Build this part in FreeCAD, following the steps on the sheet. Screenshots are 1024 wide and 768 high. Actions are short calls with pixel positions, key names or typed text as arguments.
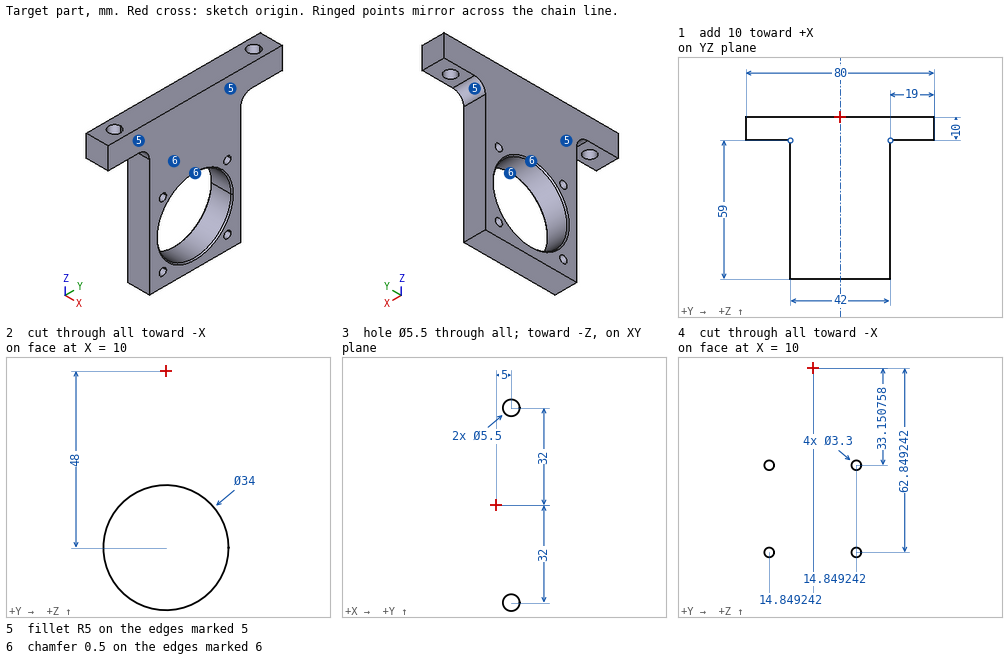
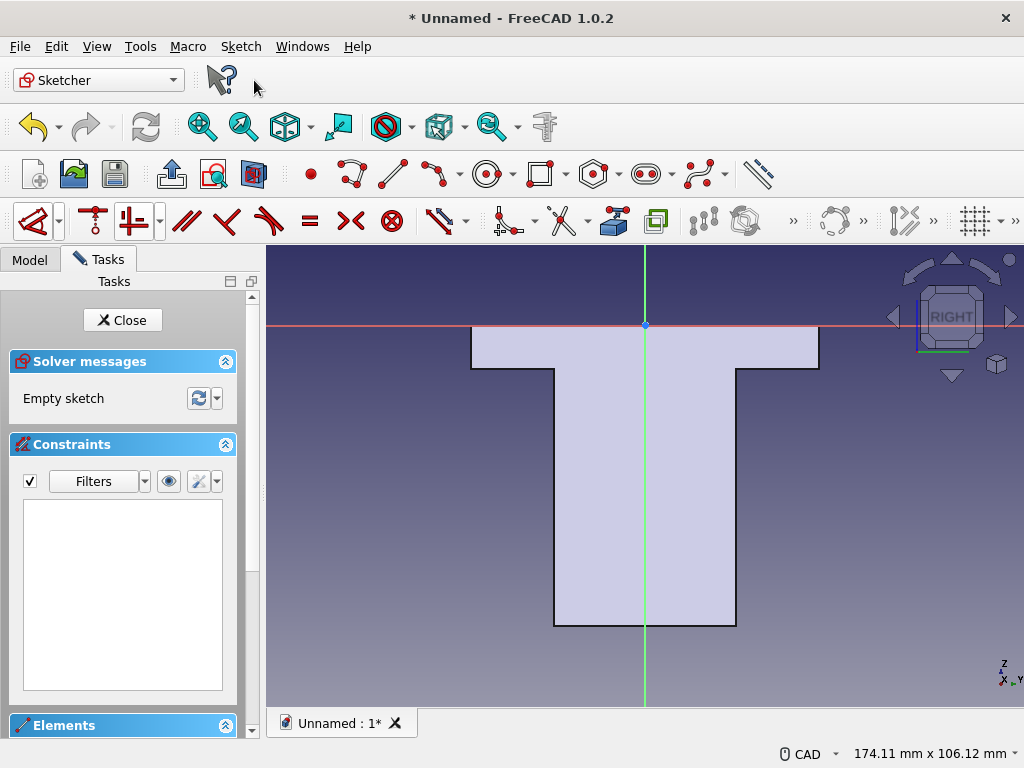
click(486, 174)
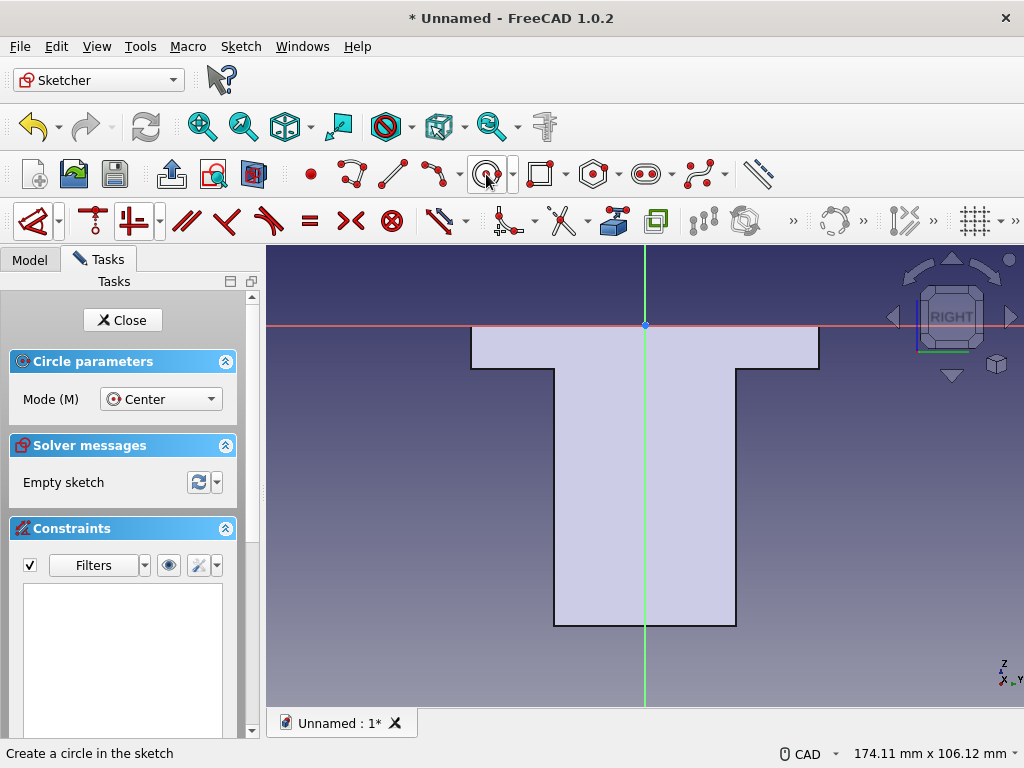
click(645, 535)
move(697, 482)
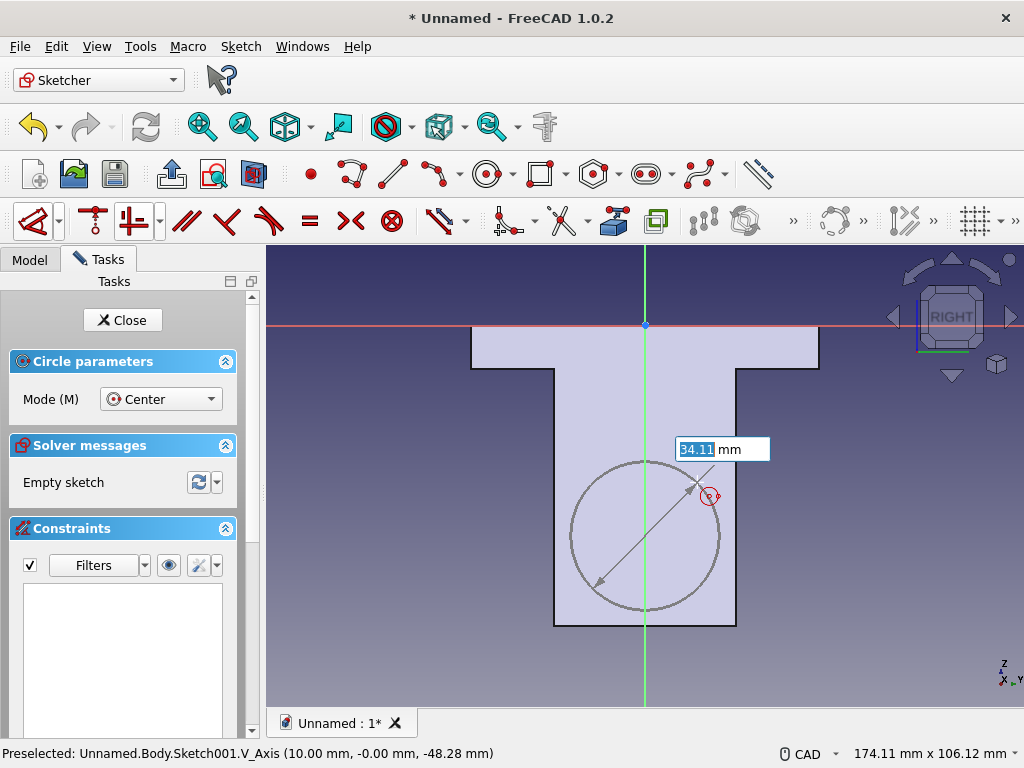
text(34)
key(Return)
key(Escape)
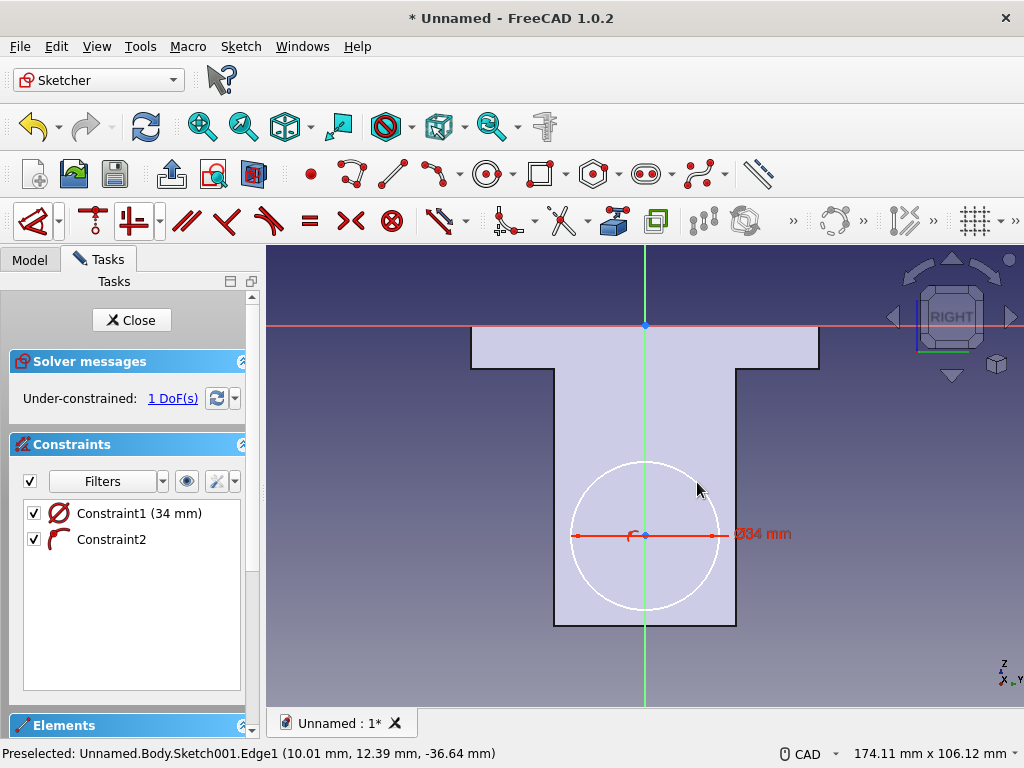
click(645, 536)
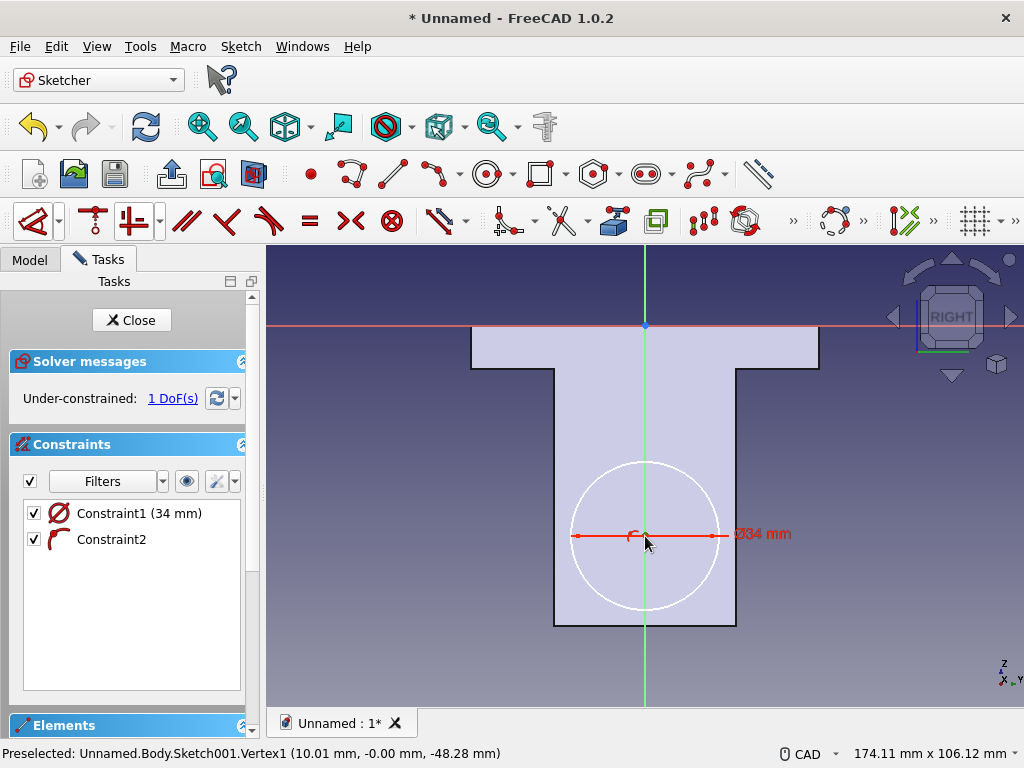
key(i)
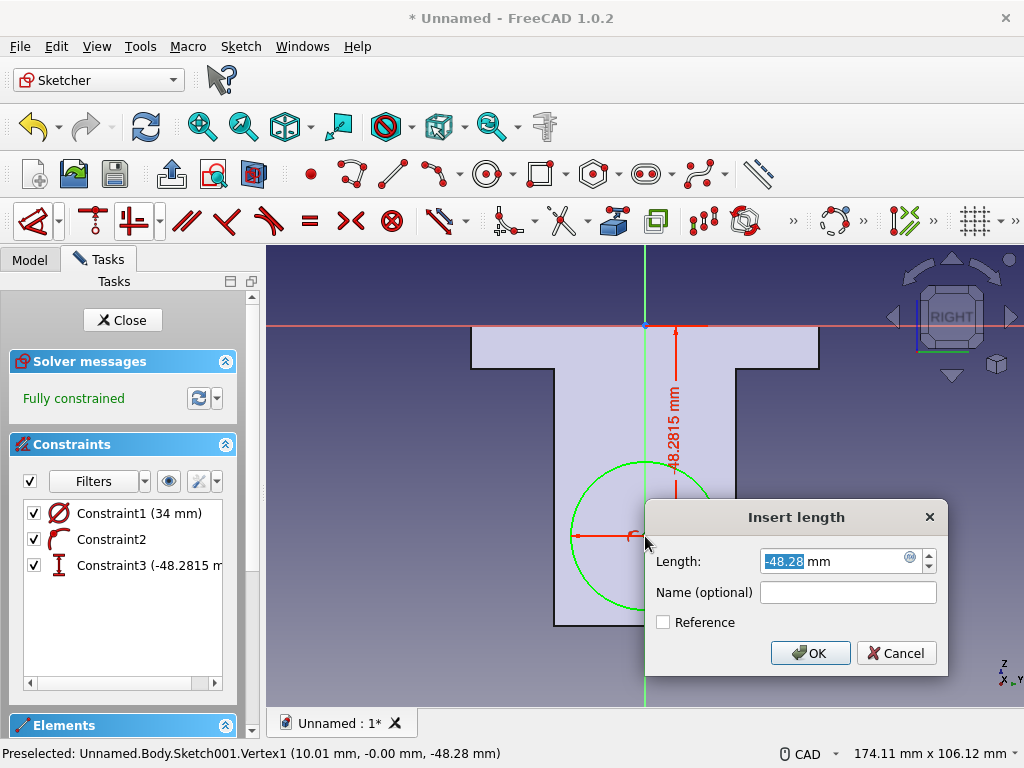
text(-48)
key(Return)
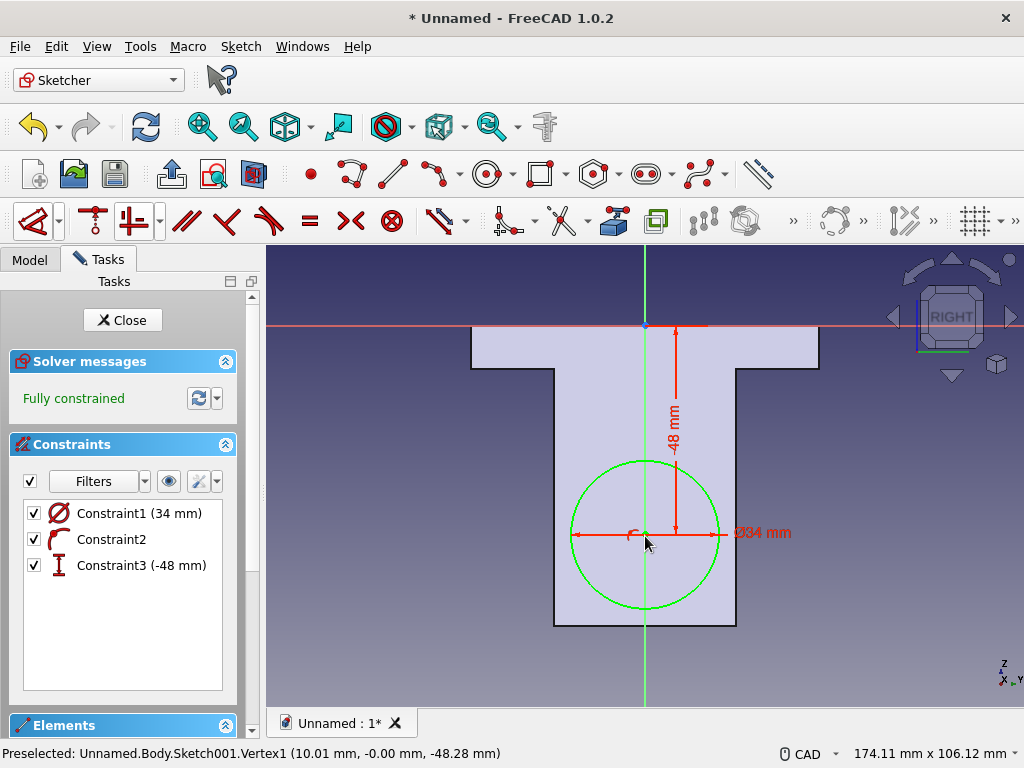
click(123, 320)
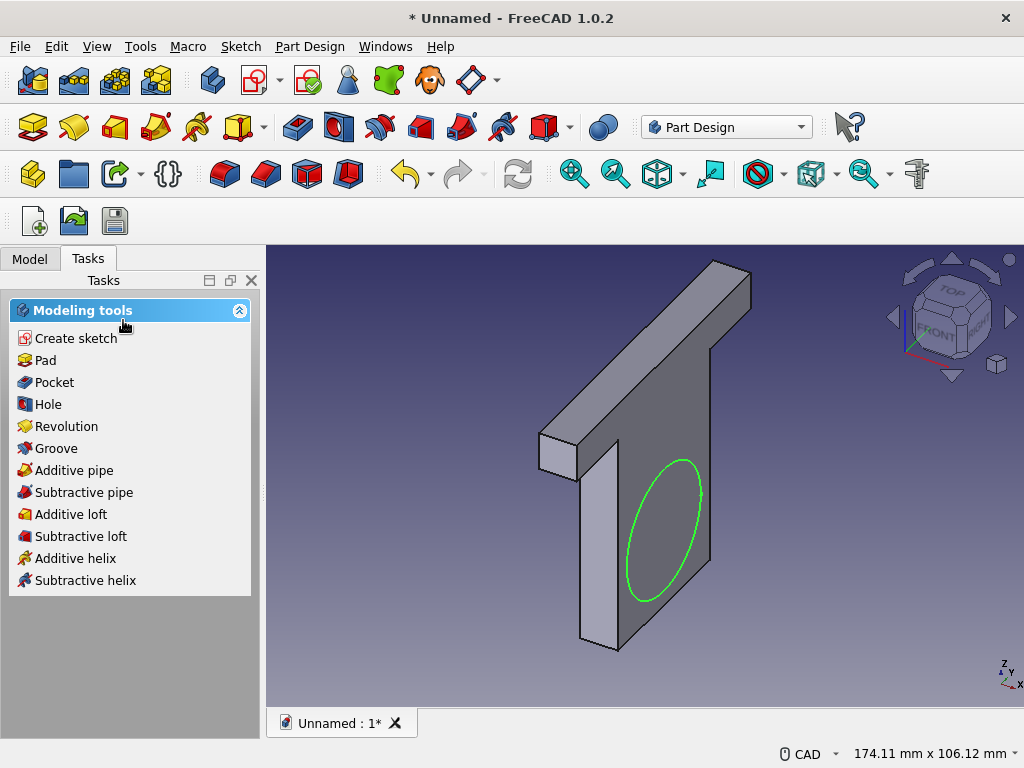
click(298, 128)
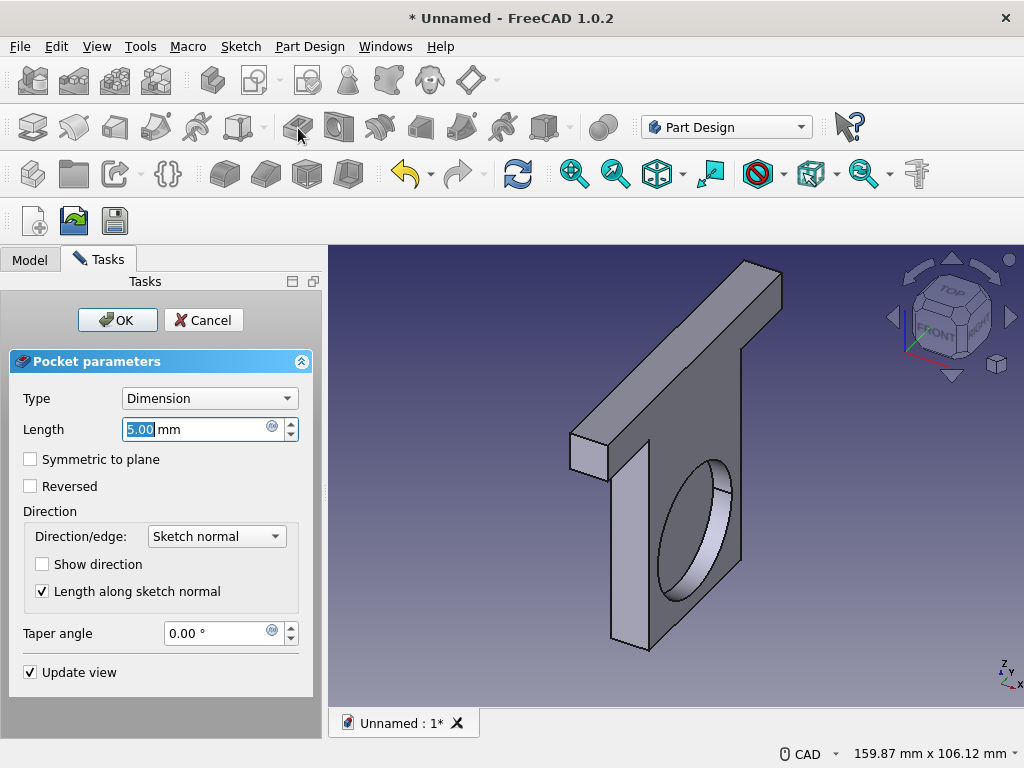
click(210, 398)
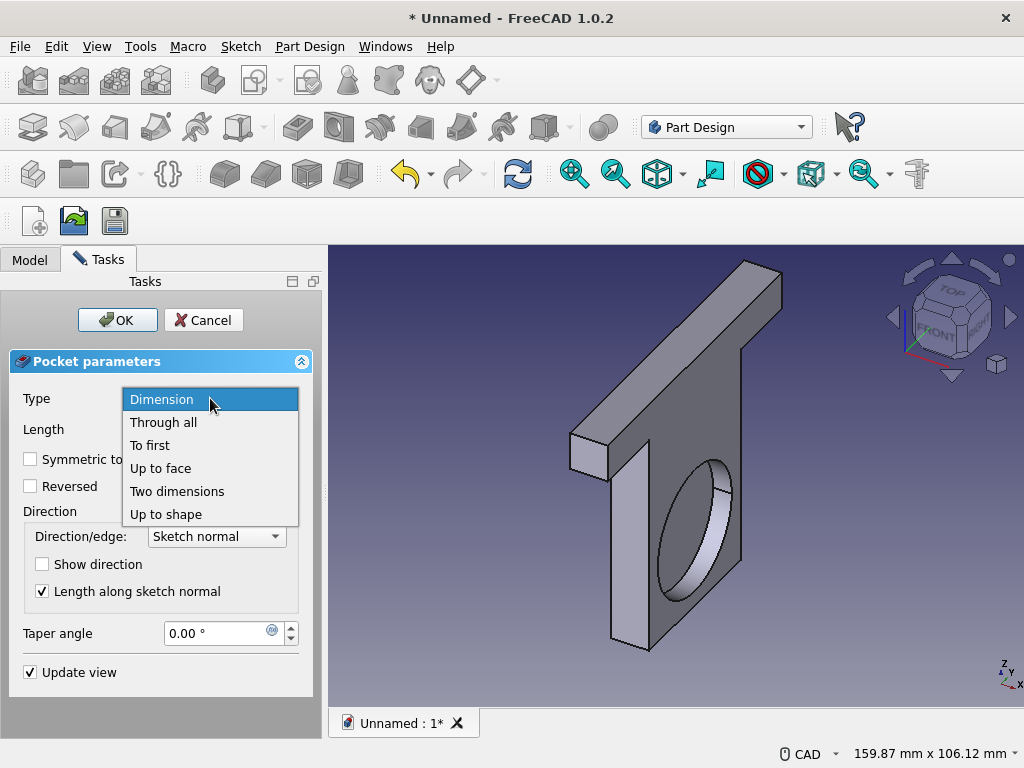
click(208, 422)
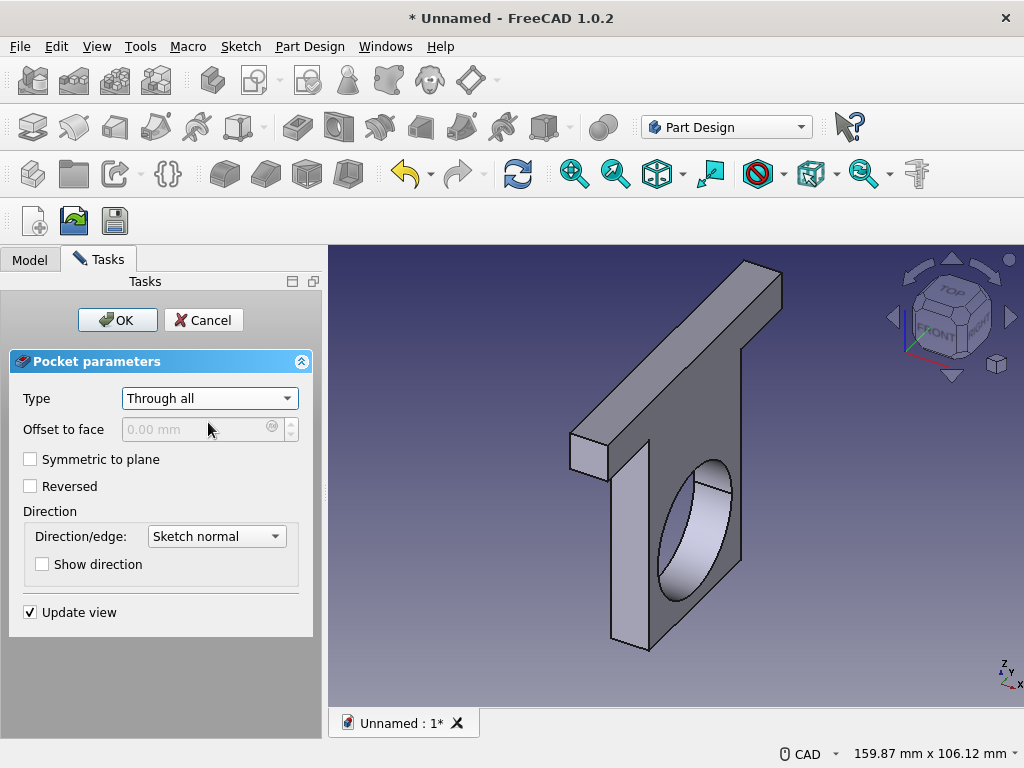
click(118, 320)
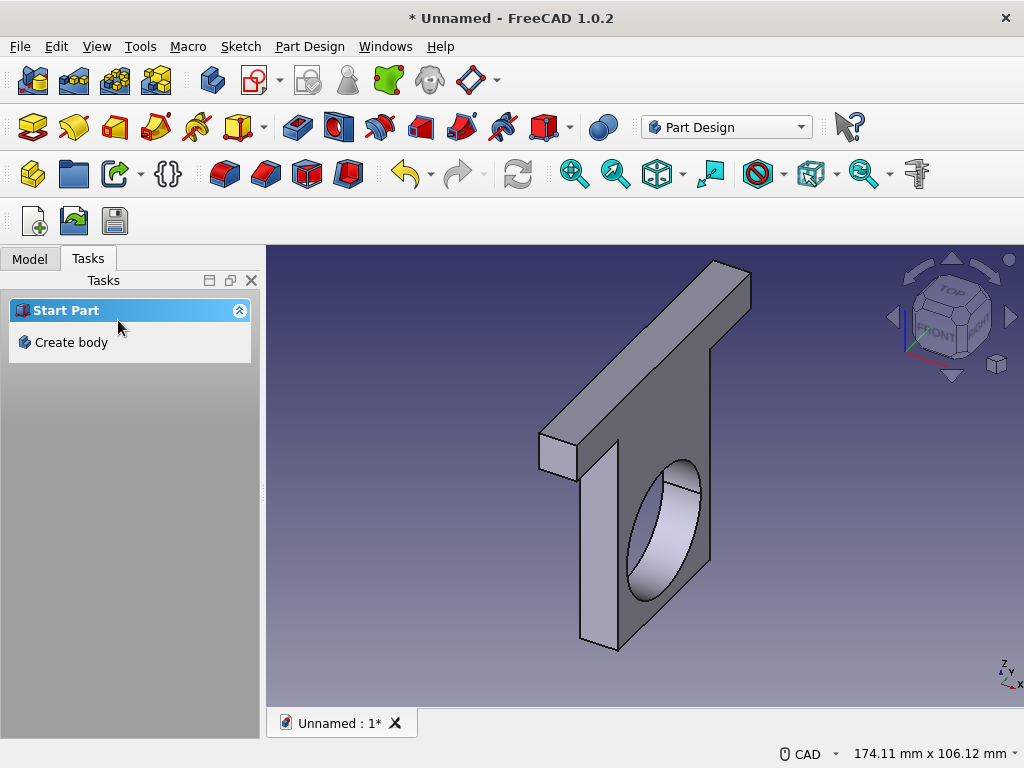
click(254, 80)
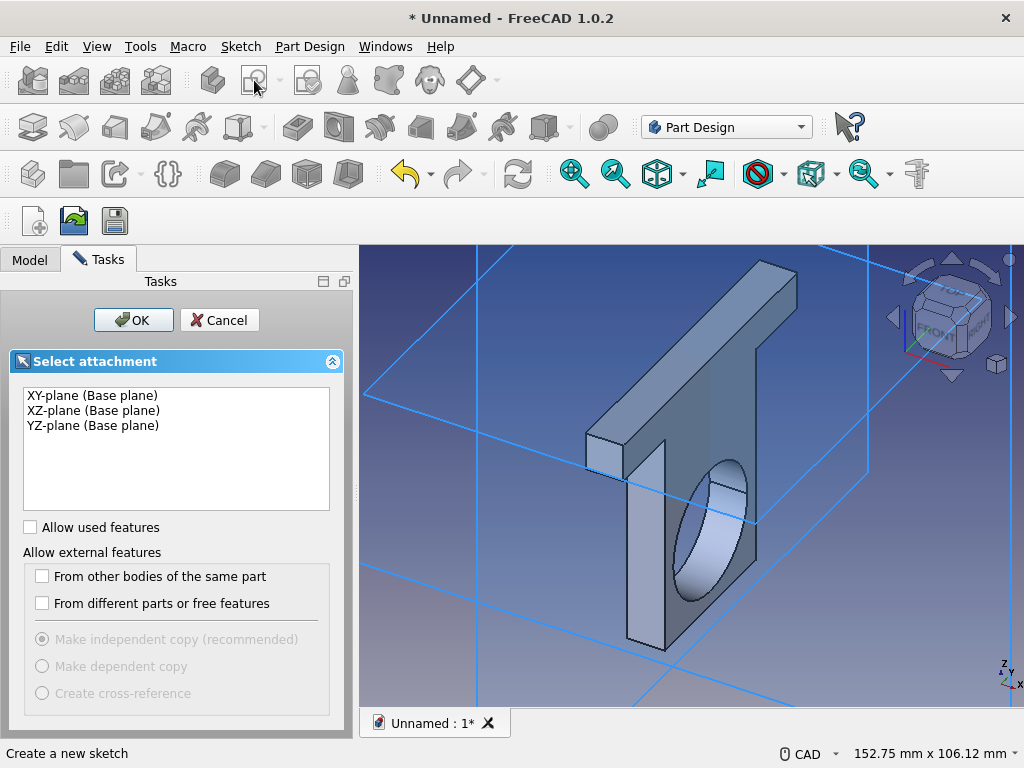
click(84, 396)